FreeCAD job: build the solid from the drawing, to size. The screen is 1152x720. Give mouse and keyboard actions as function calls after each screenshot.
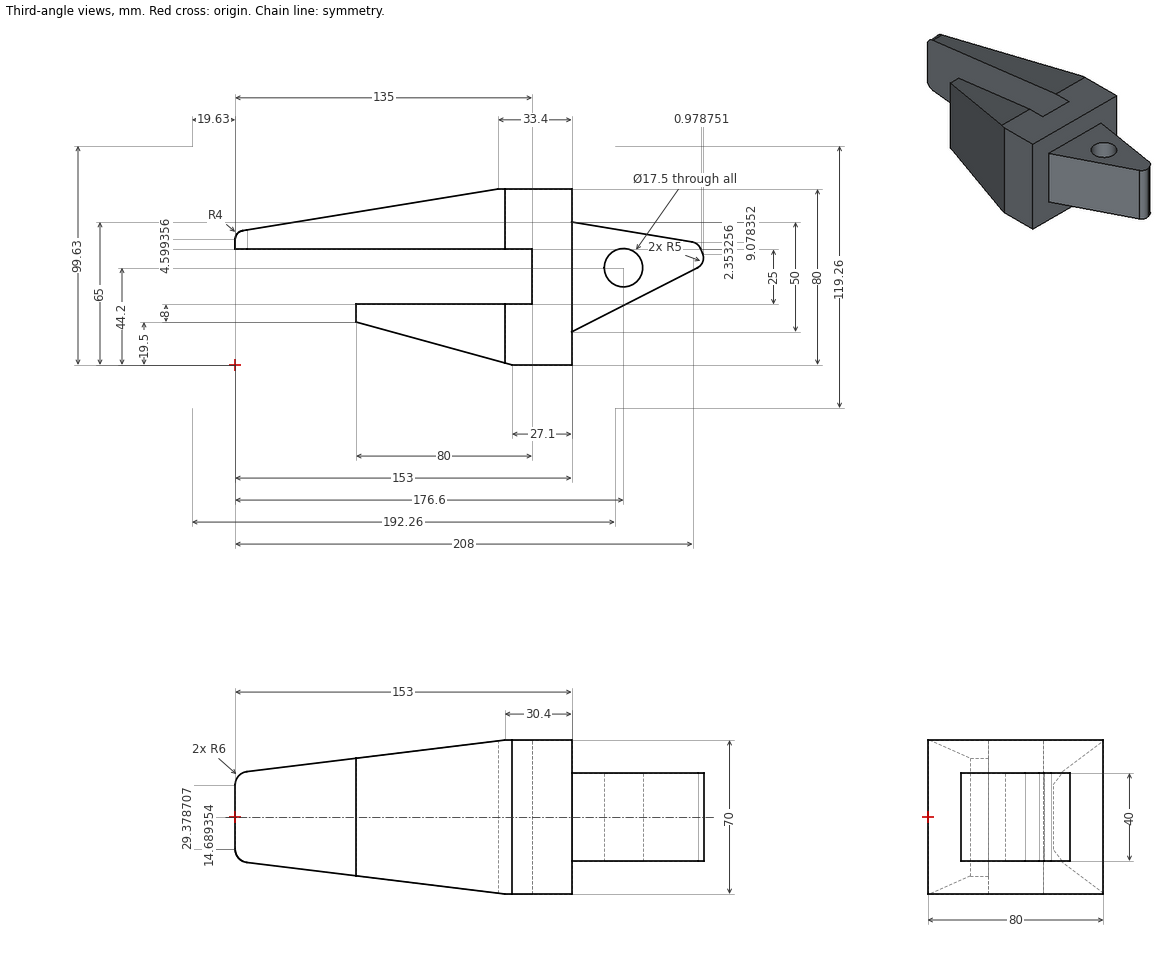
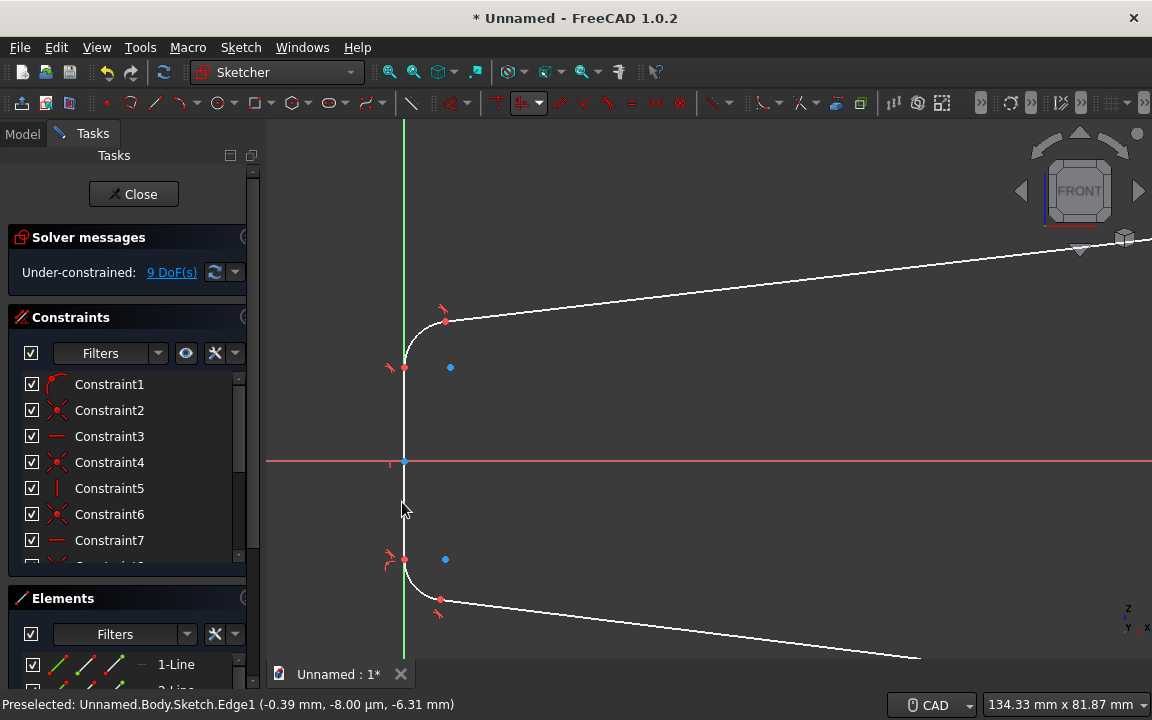
click(426, 328)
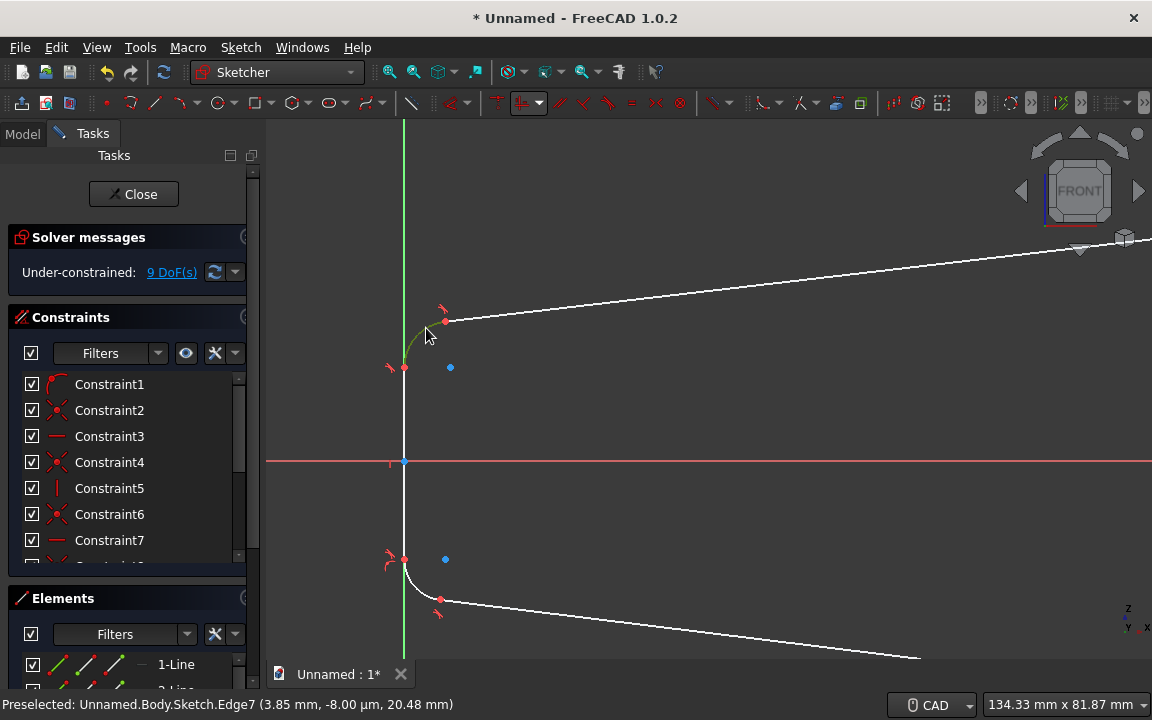
click(408, 577)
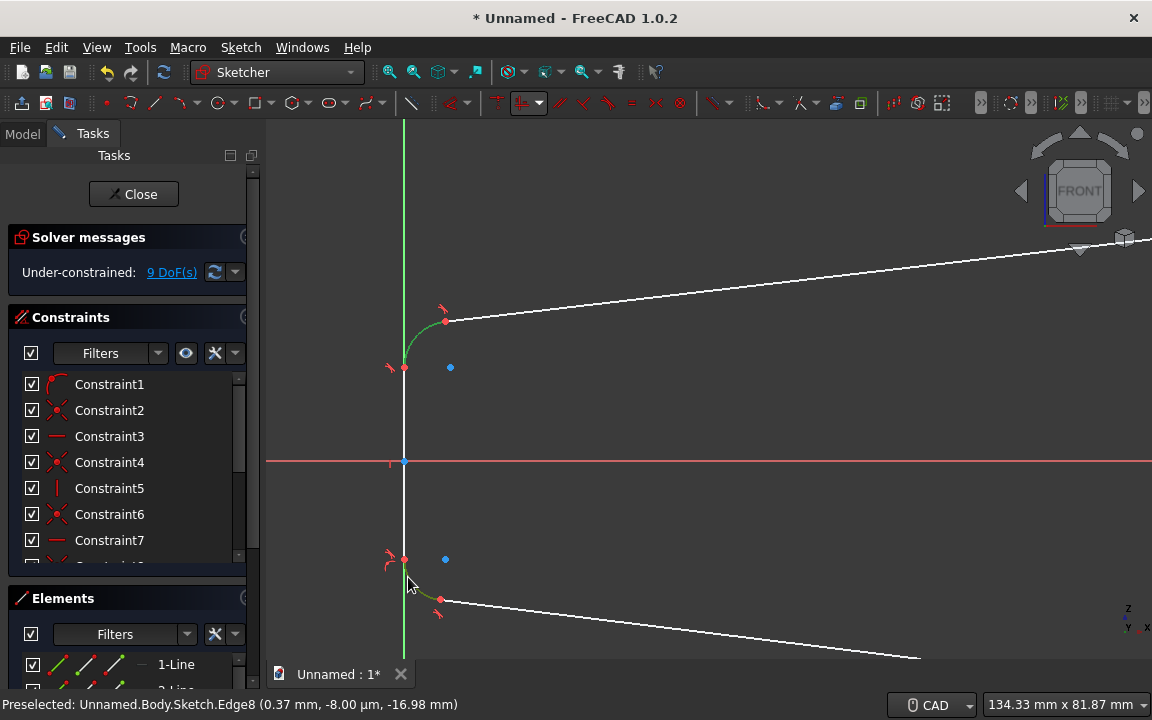
click(632, 104)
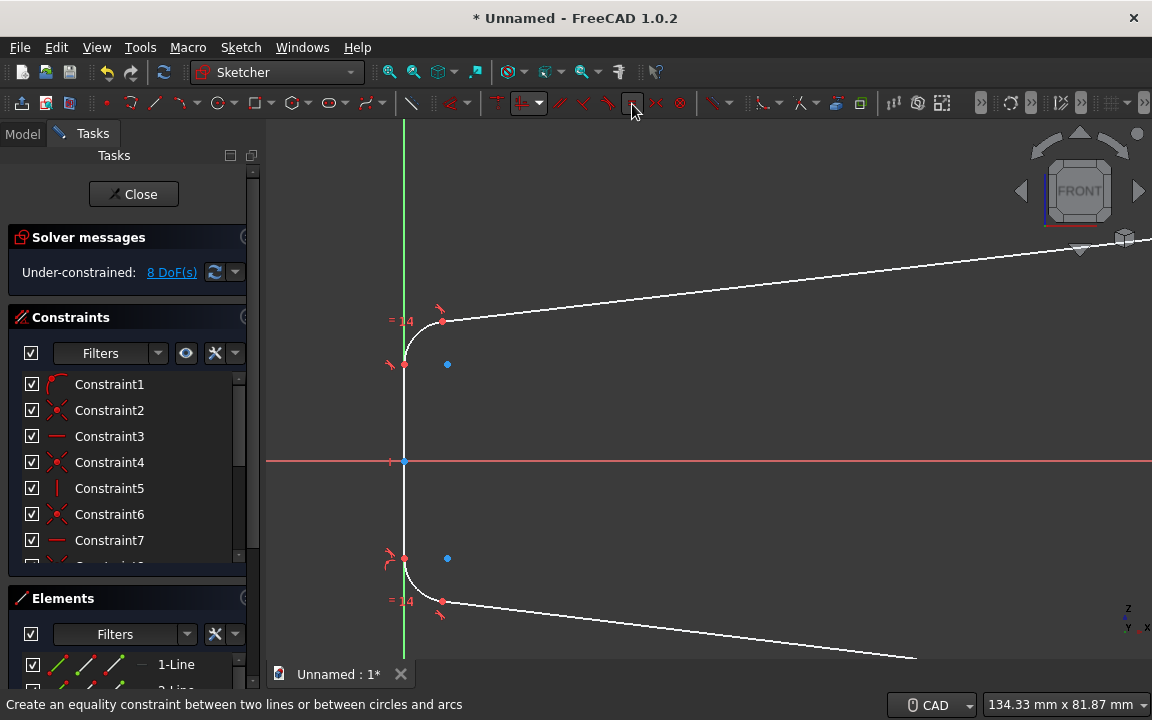
scroll(421, 330, down, 4)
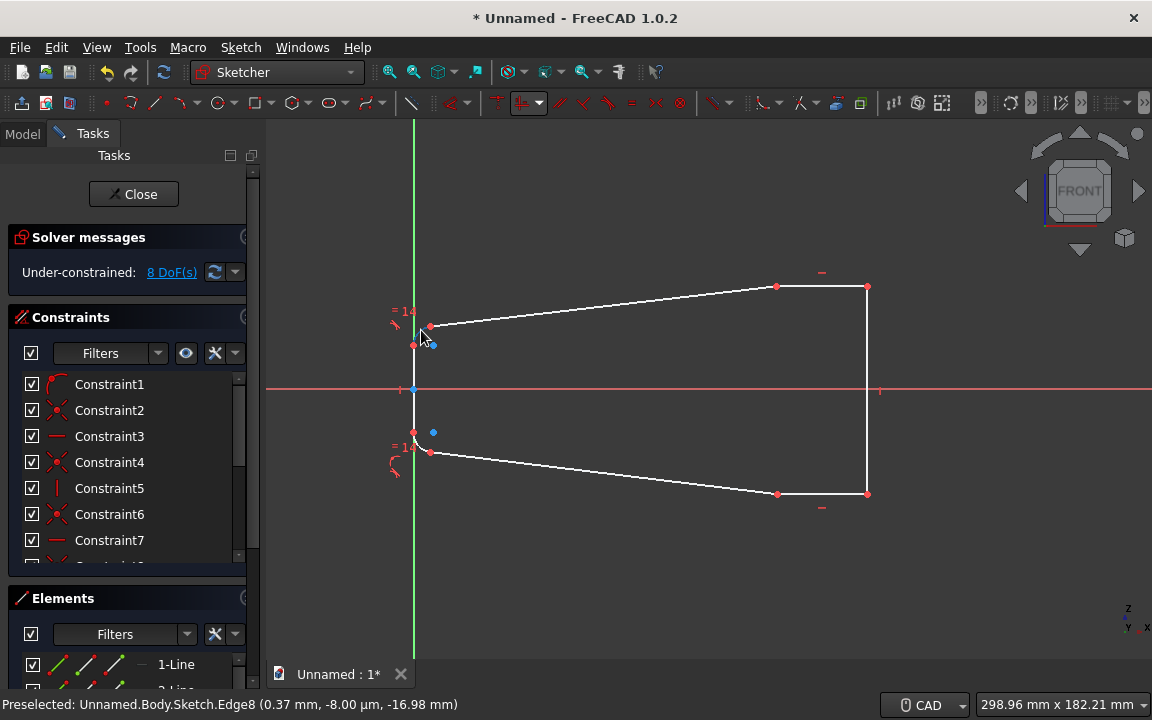
click(777, 286)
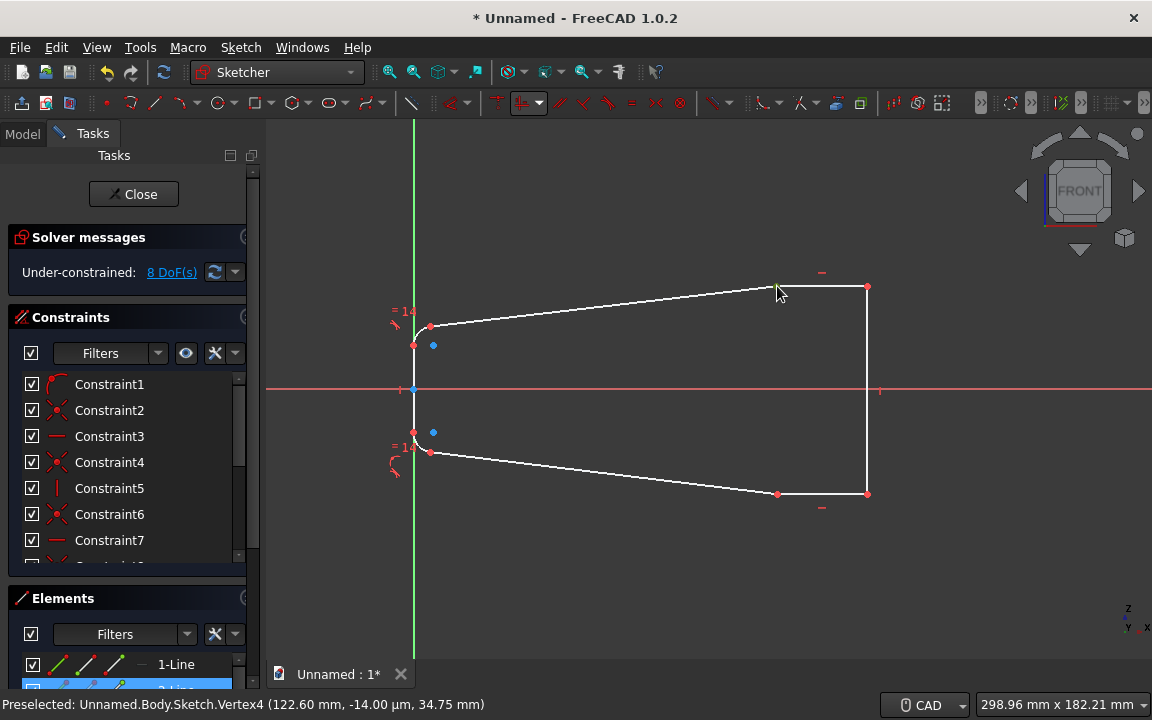
click(777, 494)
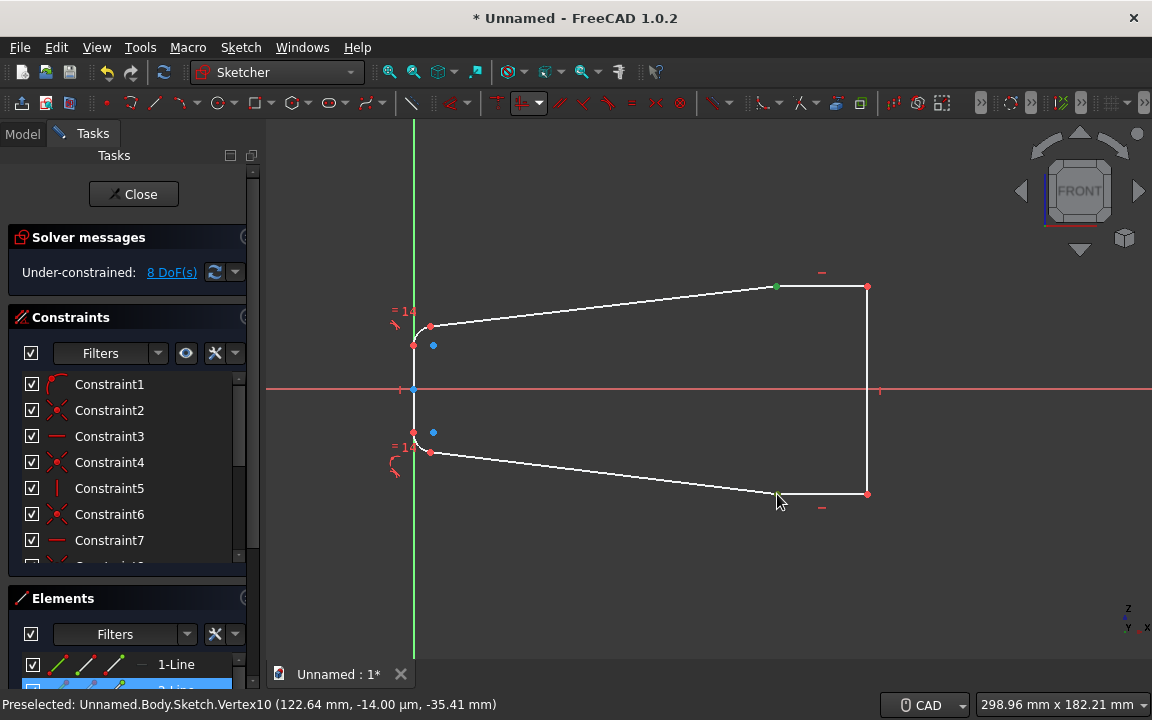
click(344, 389)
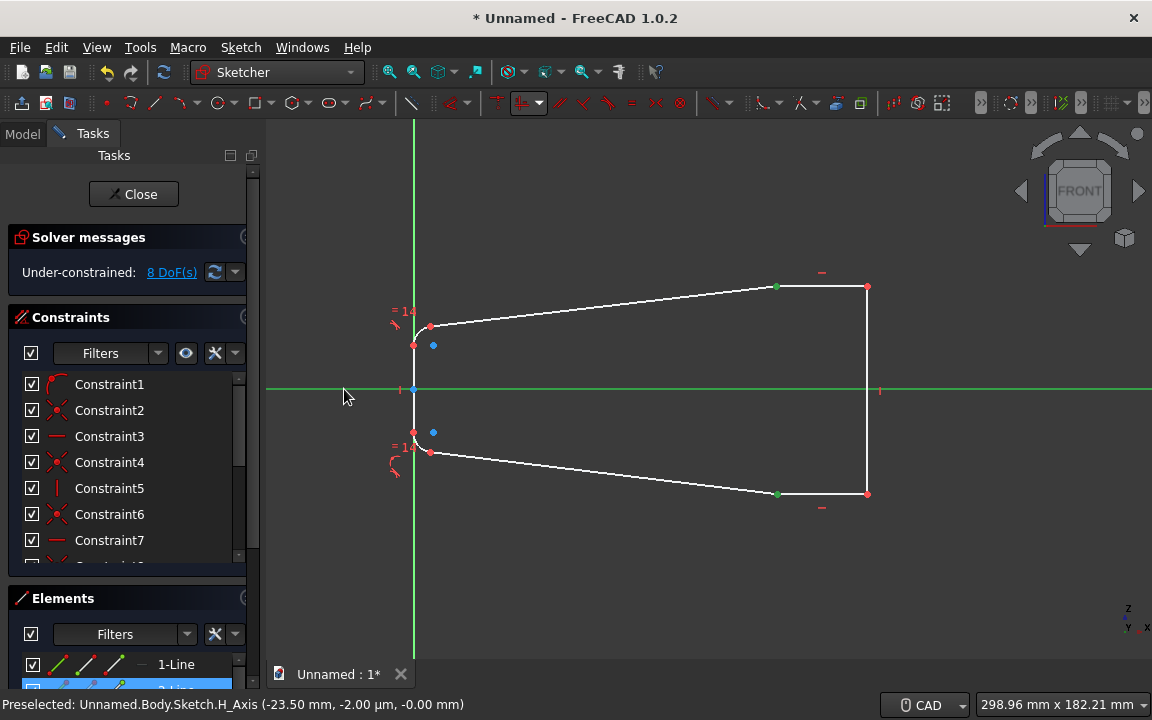
click(656, 104)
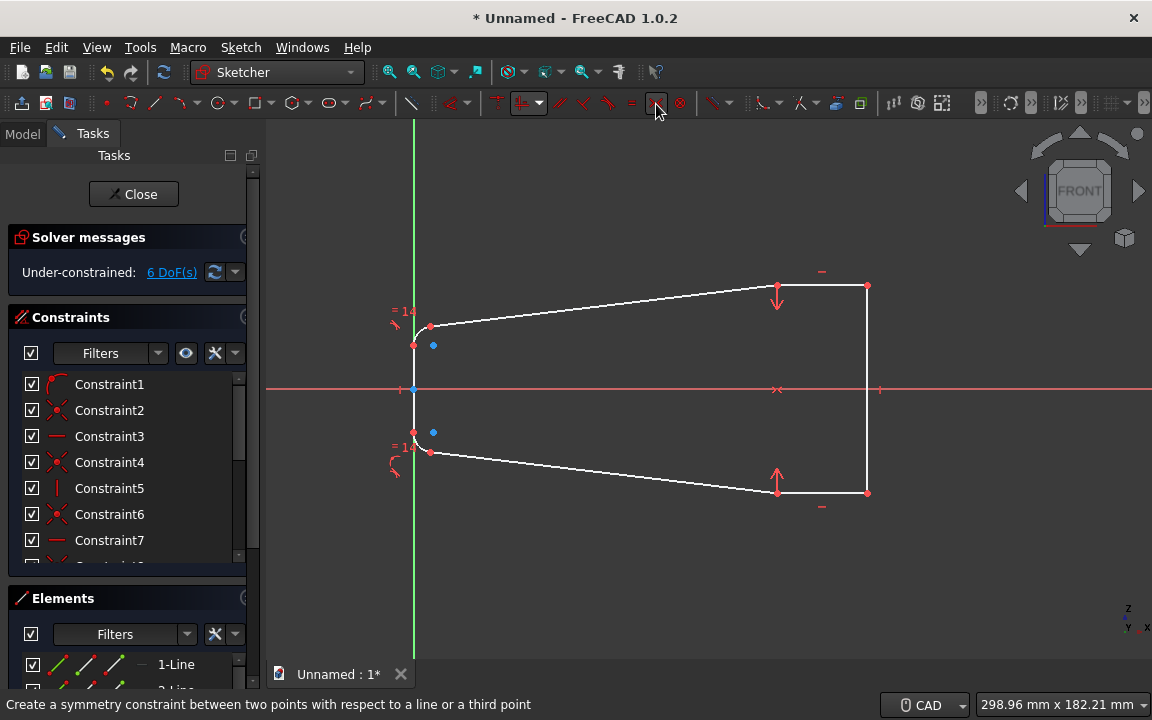
click(450, 104)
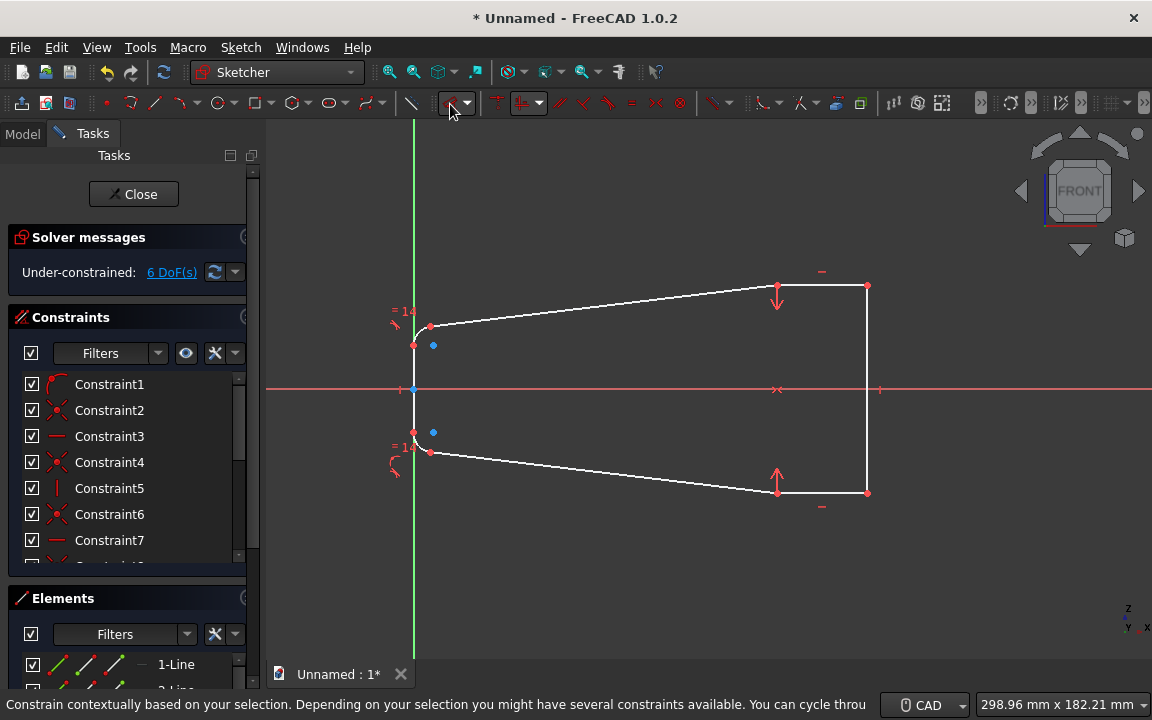
scroll(415, 338, up, 5)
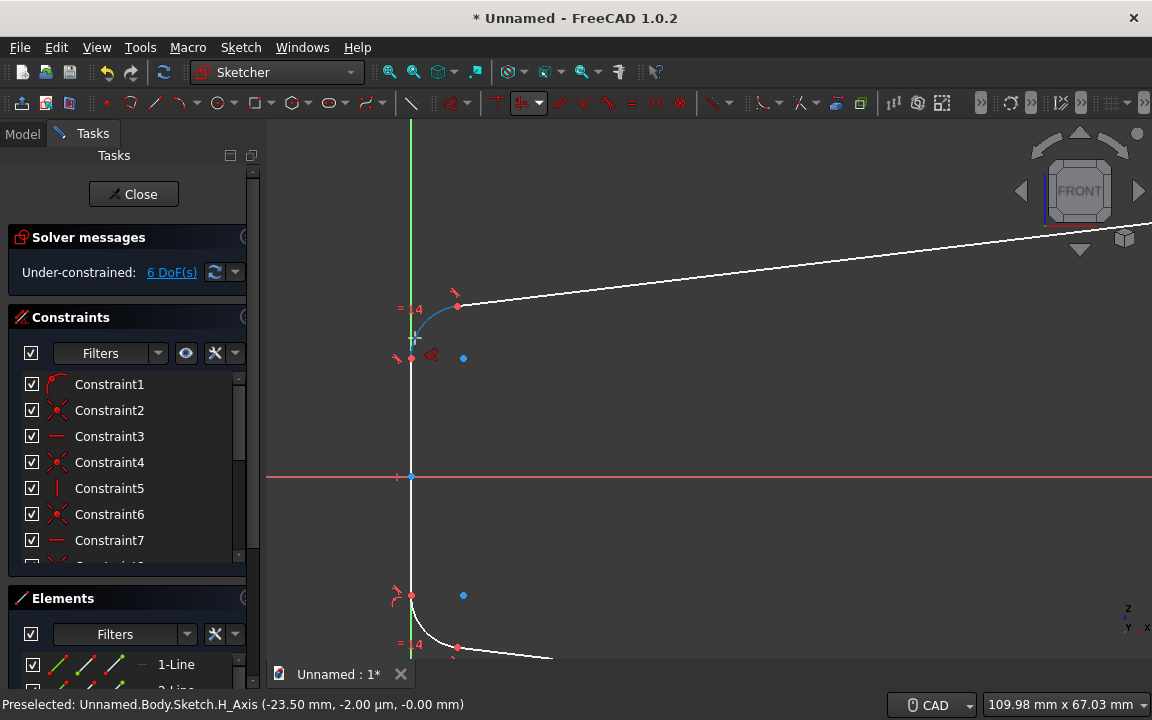
click(416, 336)
click(387, 322)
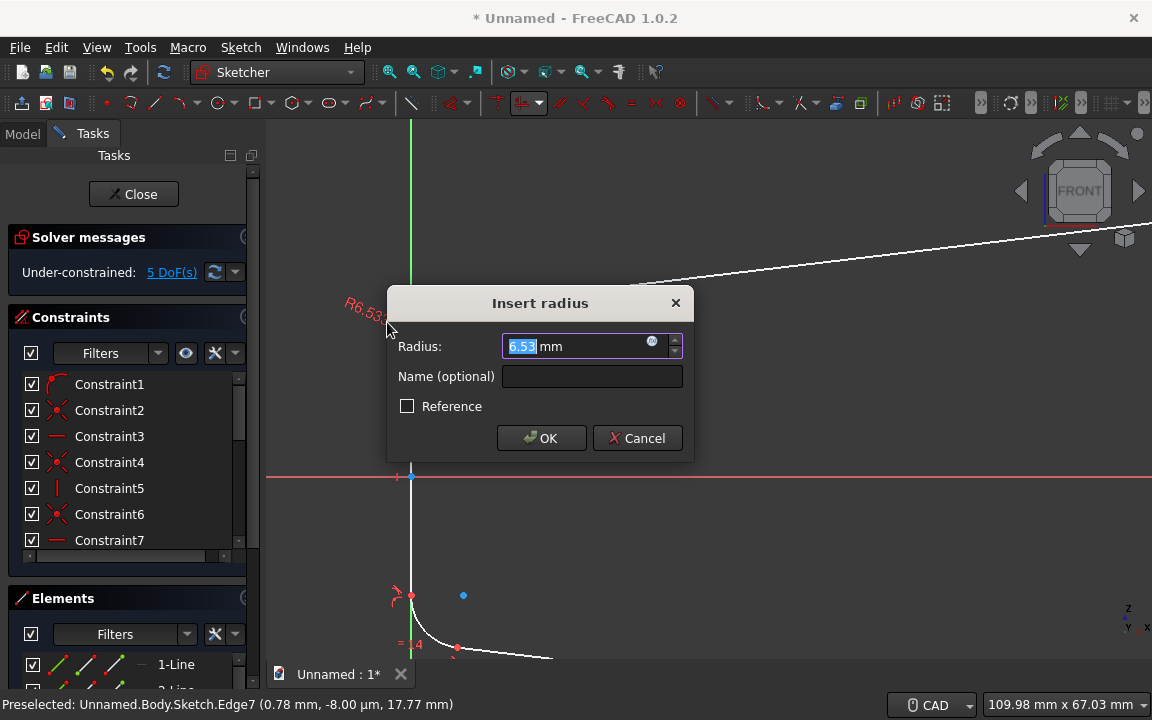
text(6)
key(Return)